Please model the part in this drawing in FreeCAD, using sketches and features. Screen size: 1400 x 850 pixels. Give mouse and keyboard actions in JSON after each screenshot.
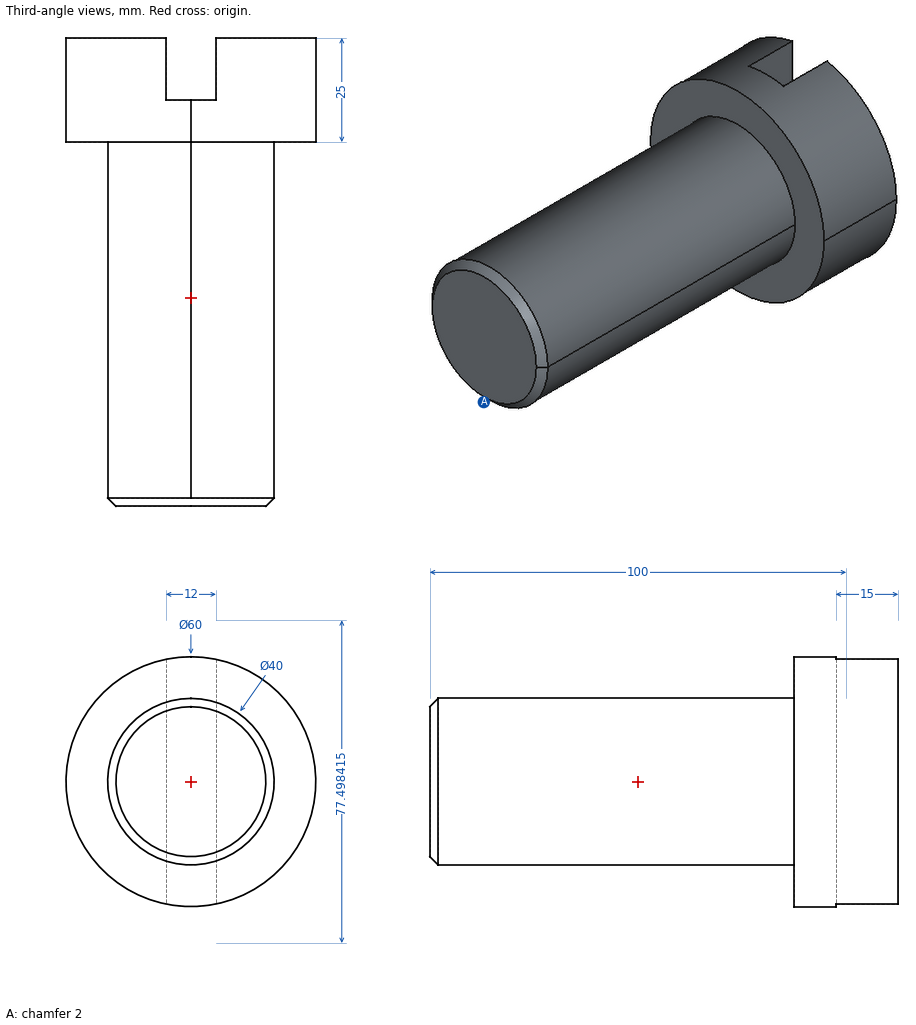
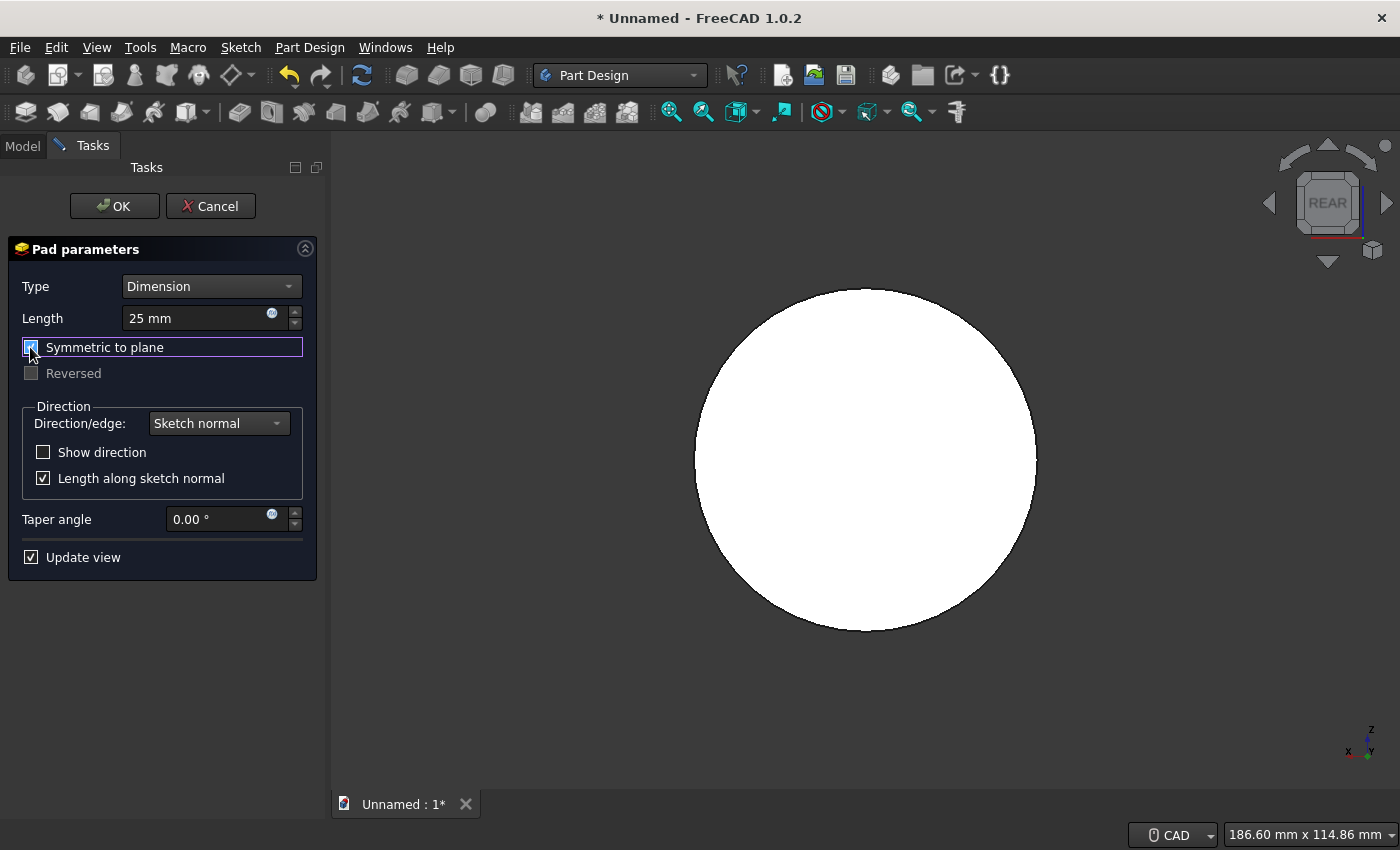
{"action": "left_click", "coordinate": [115, 206]}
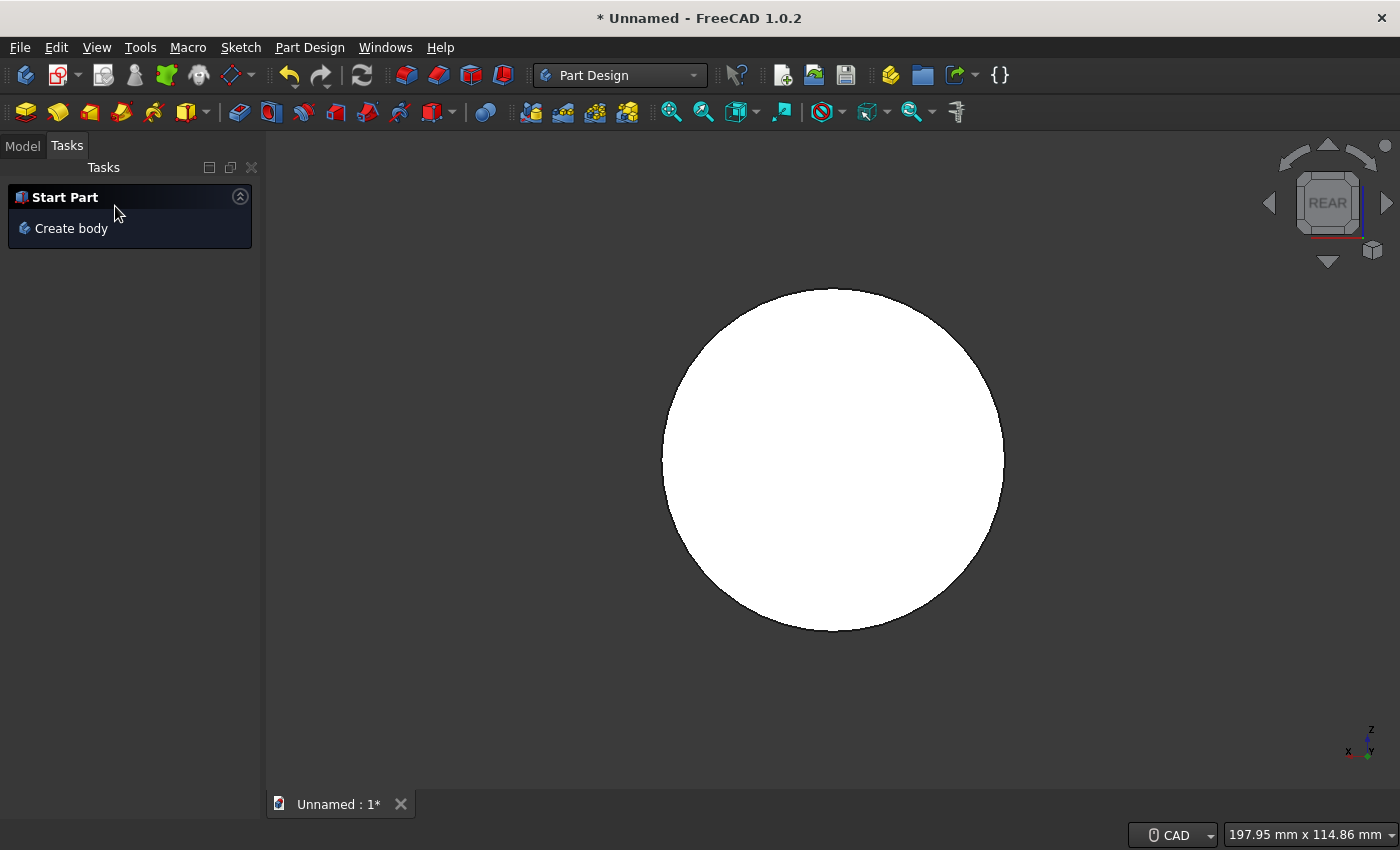
{"action": "key", "text": "0"}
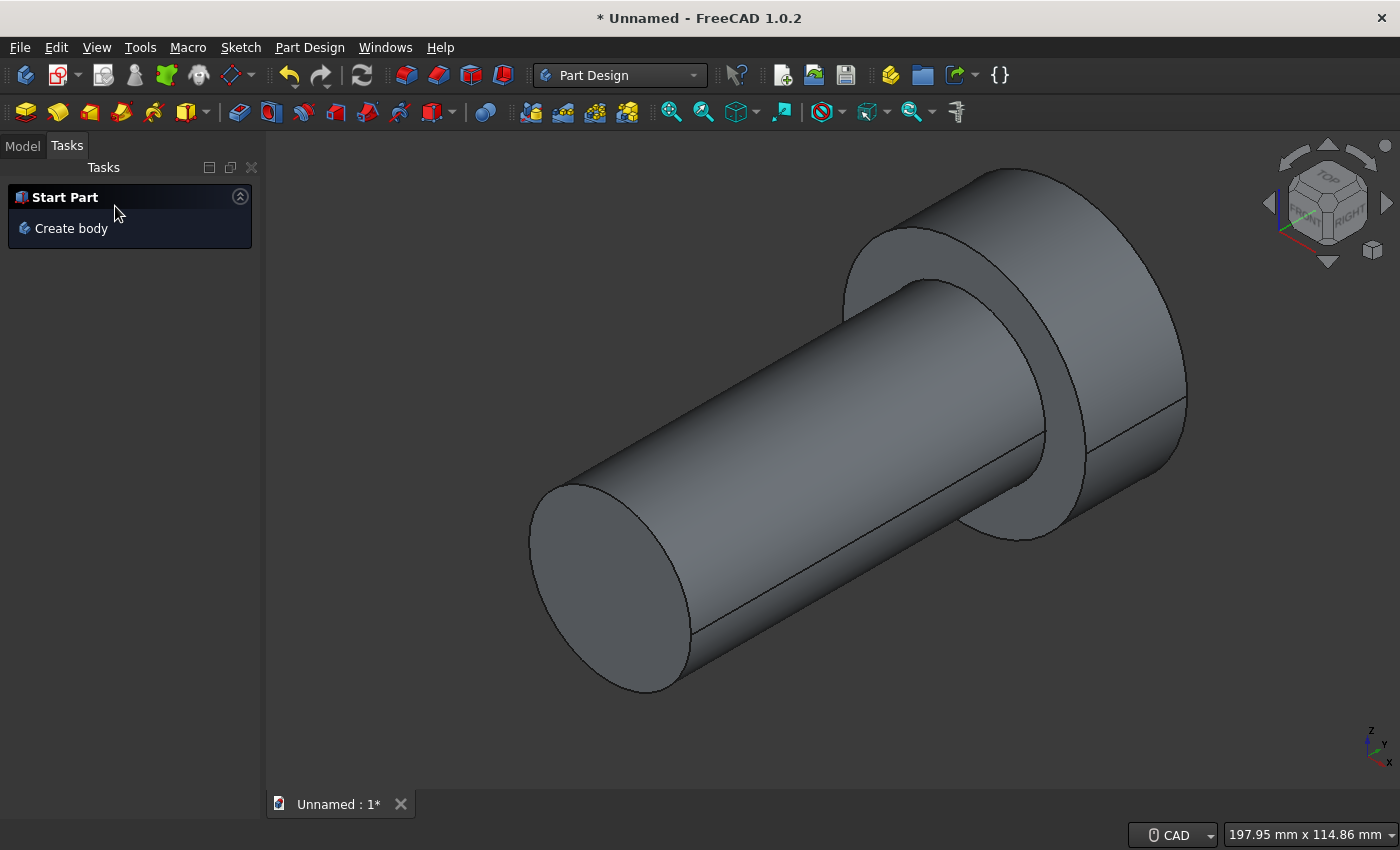
{"action": "left_click", "coordinate": [672, 112]}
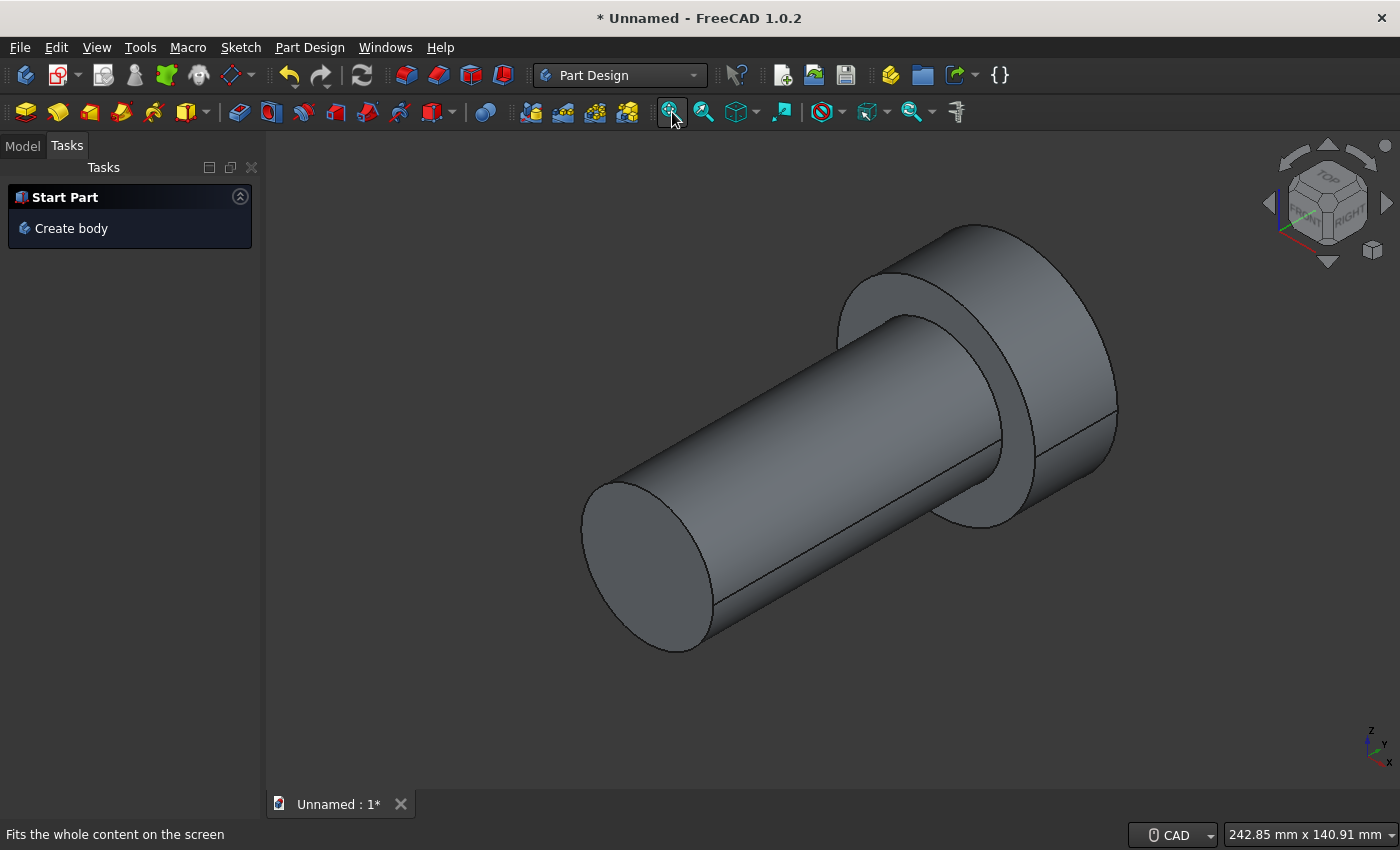
{"action": "left_click", "coordinate": [627, 482]}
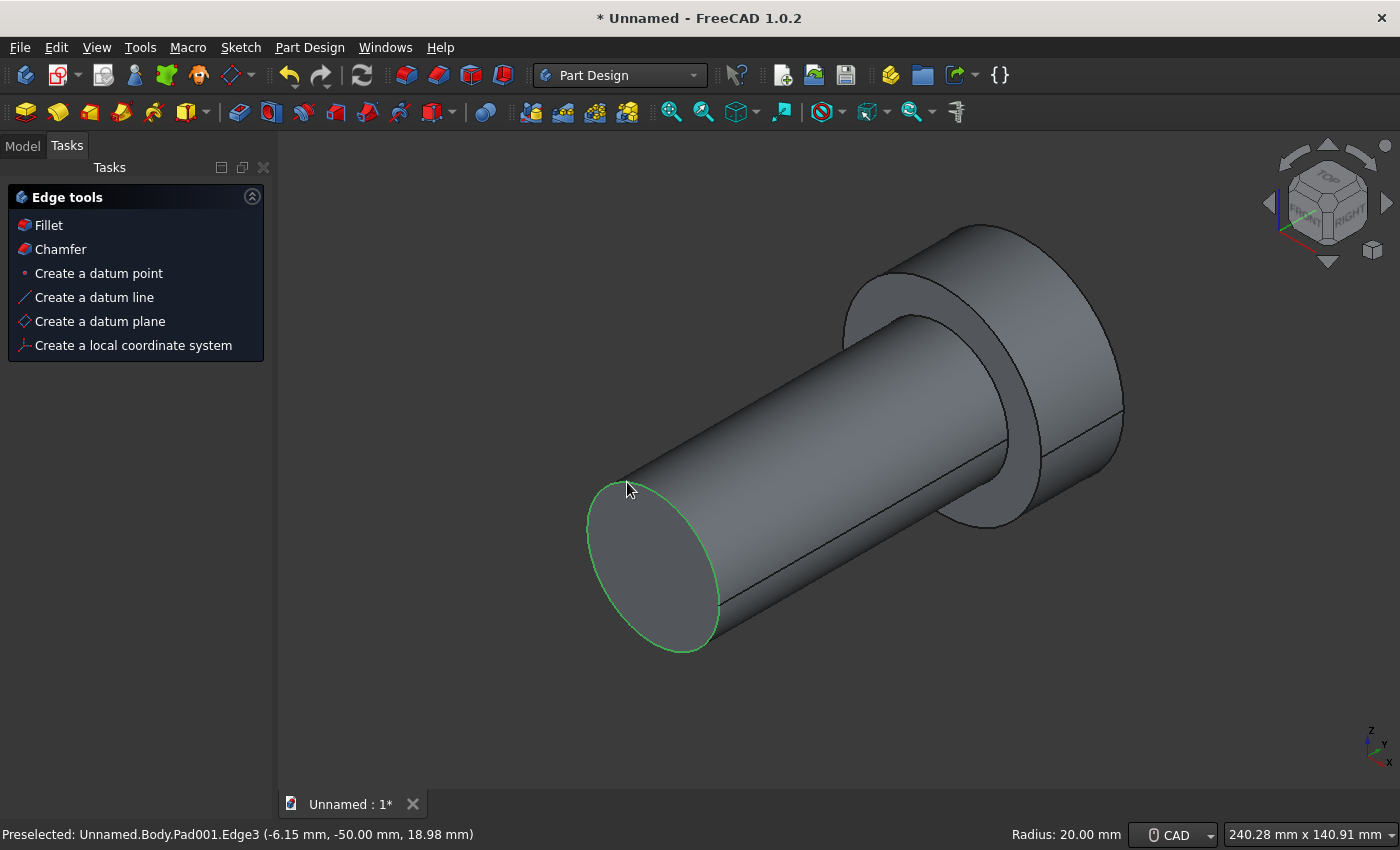
{"action": "left_click", "coordinate": [440, 76]}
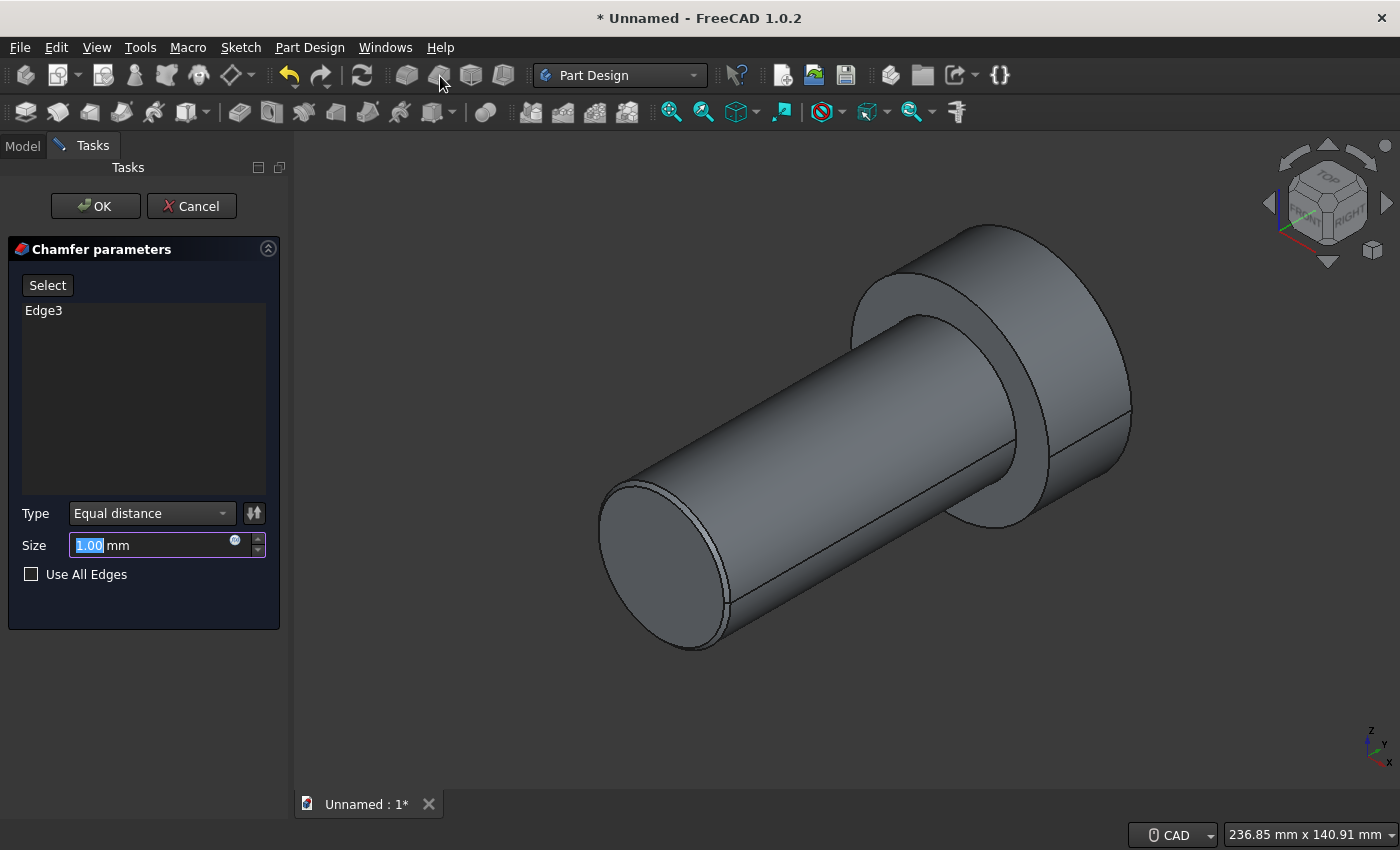
{"action": "type", "text": "2"}
{"action": "key", "text": "Tab"}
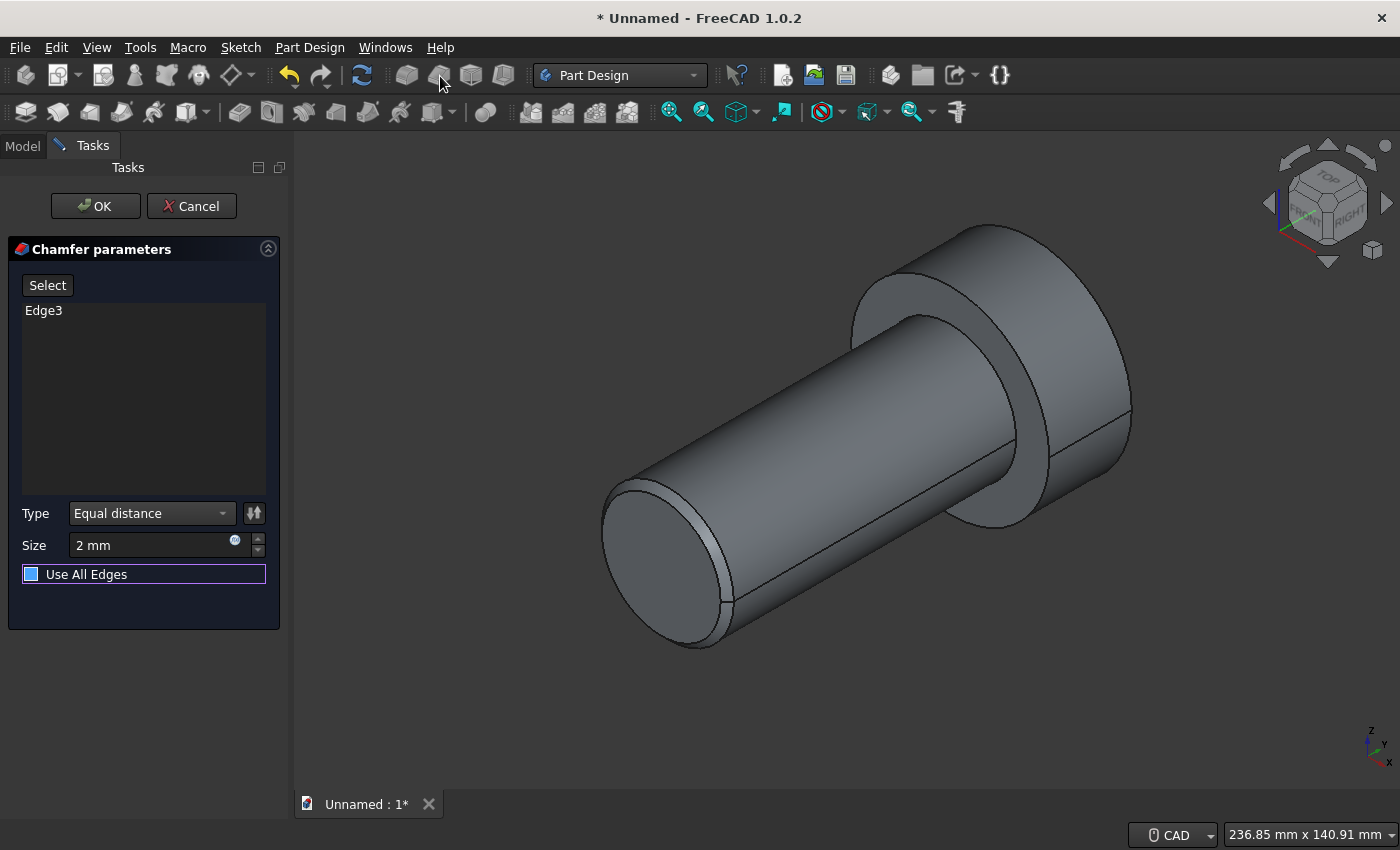
{"action": "left_click", "coordinate": [96, 206]}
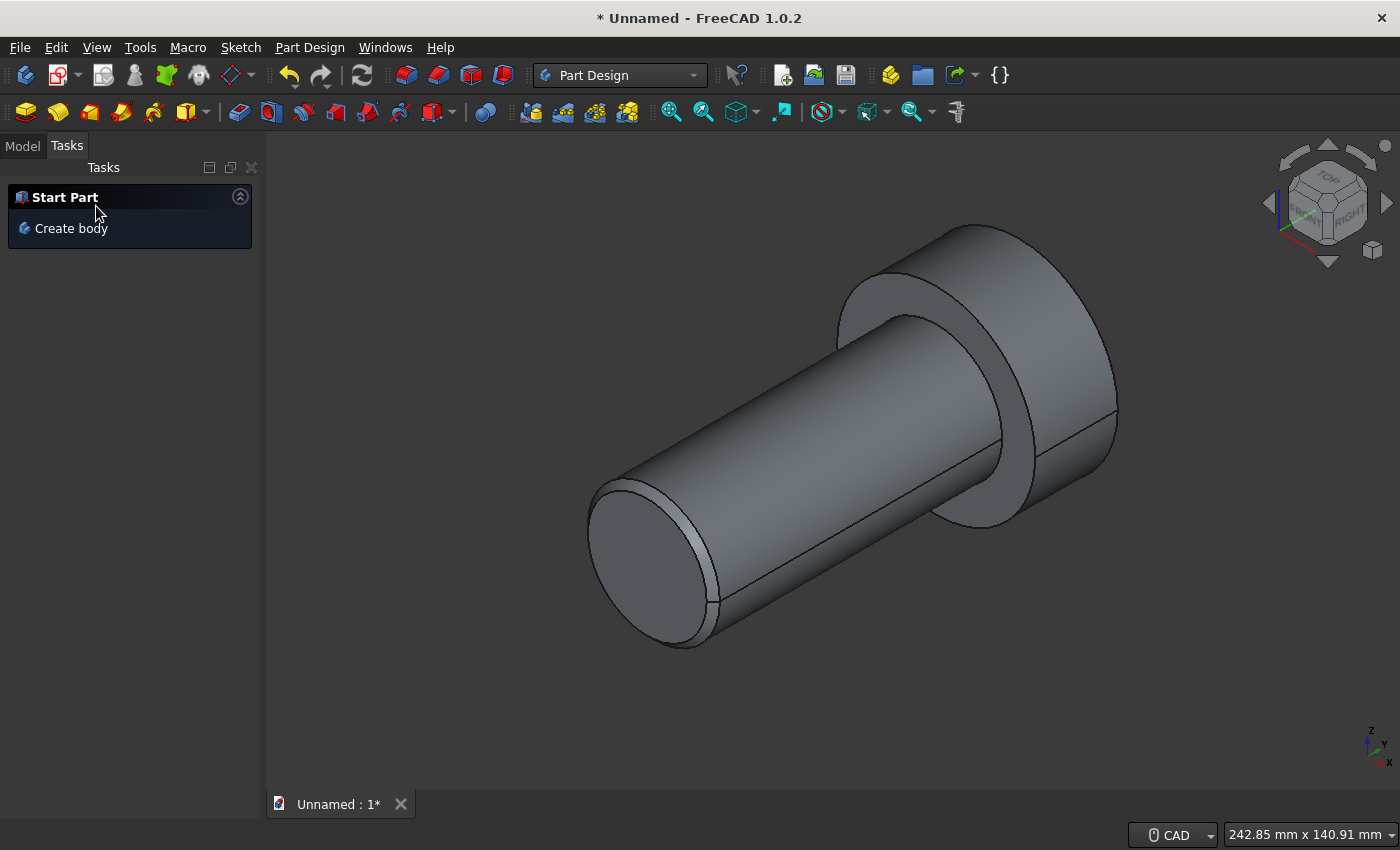
{"action": "key", "text": "4"}